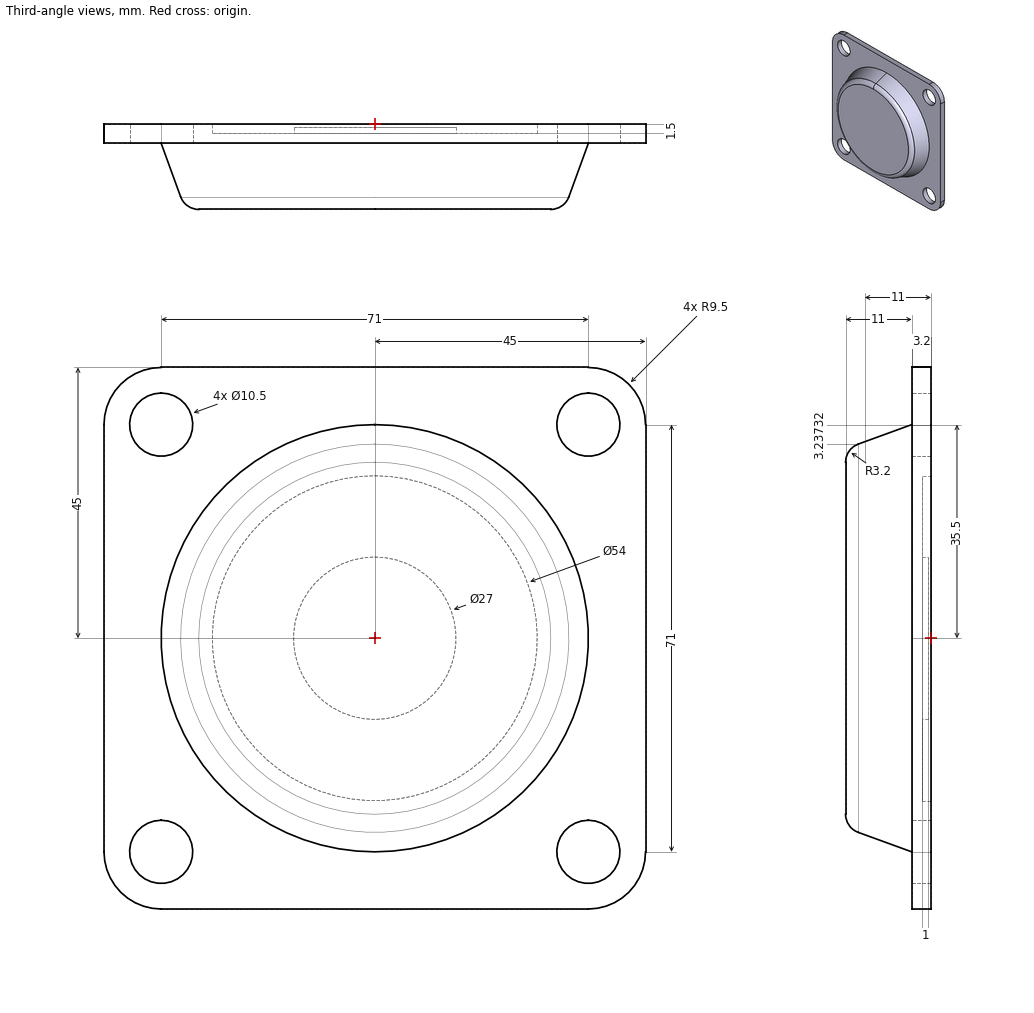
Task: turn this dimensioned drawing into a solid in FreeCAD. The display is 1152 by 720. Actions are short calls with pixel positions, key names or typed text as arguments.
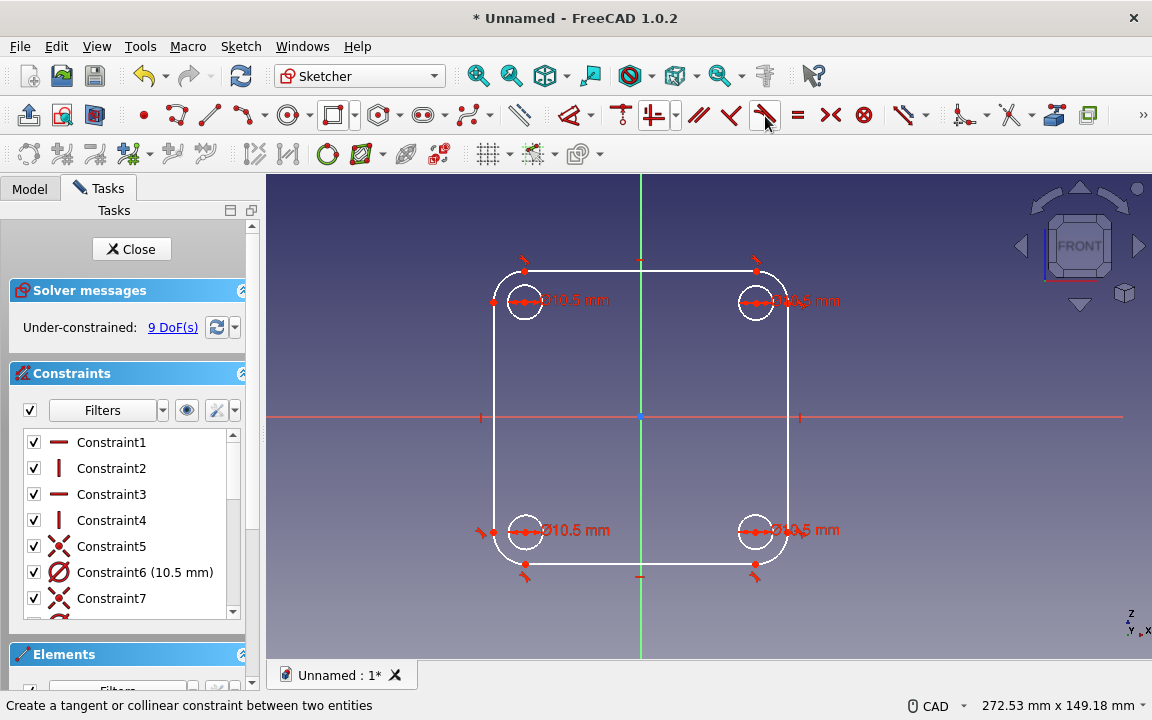
click(494, 463)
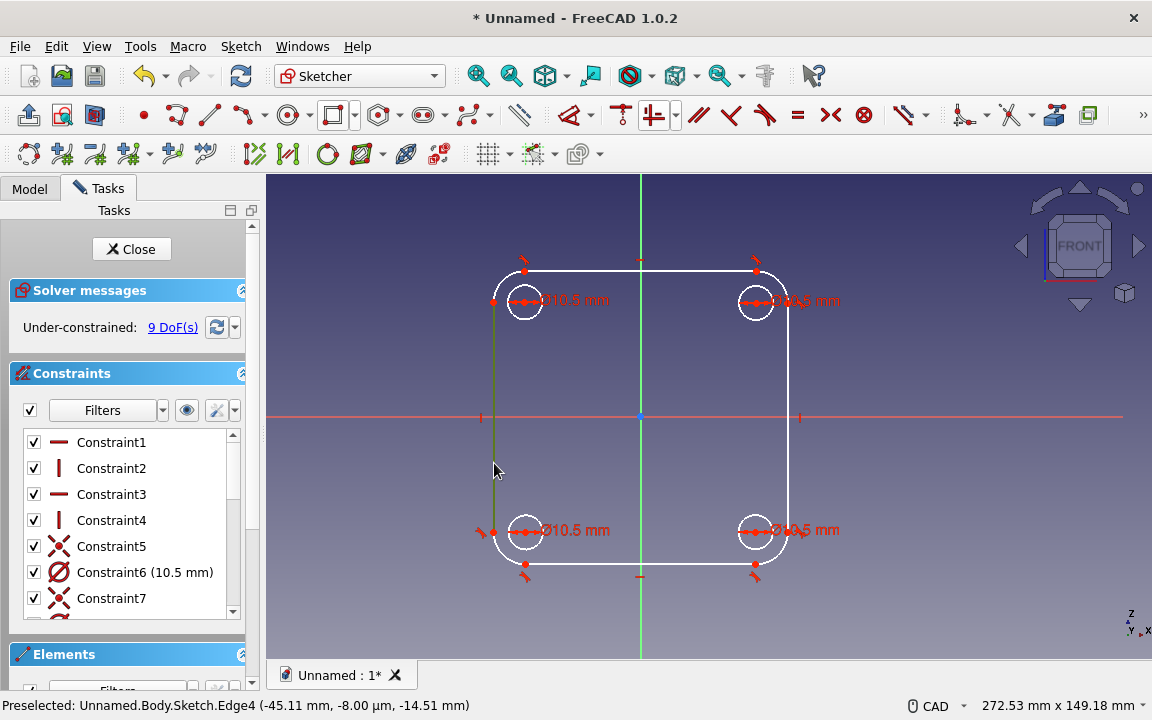
click(511, 275)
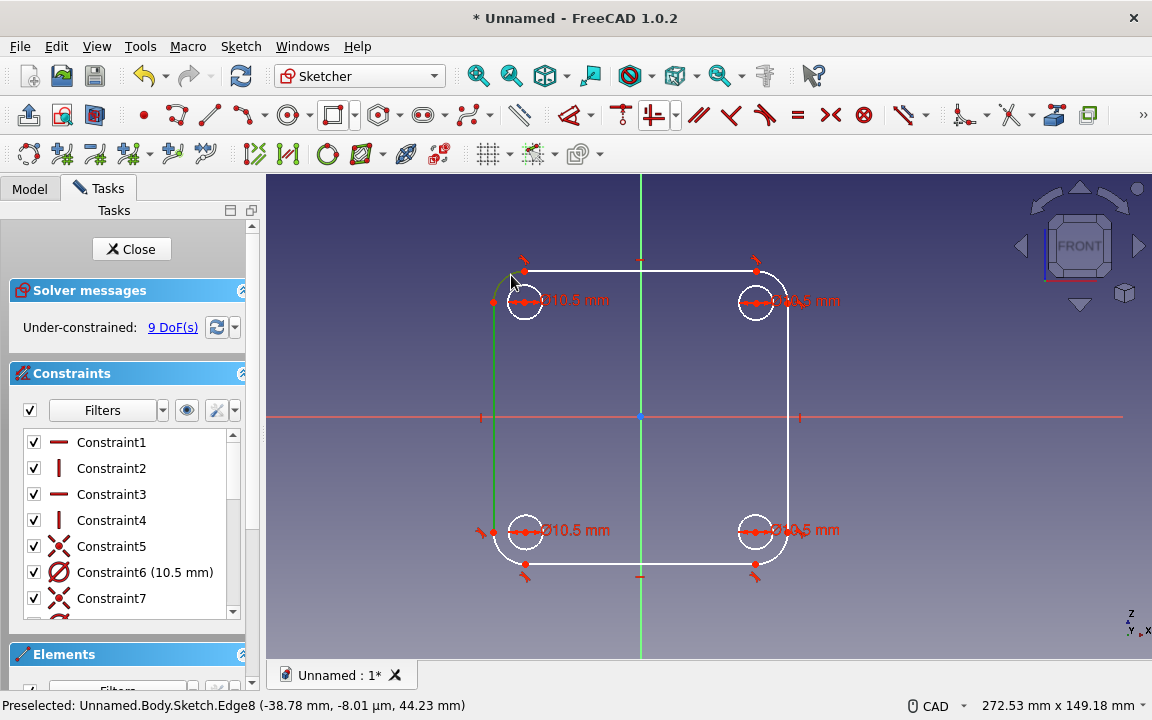
key(t)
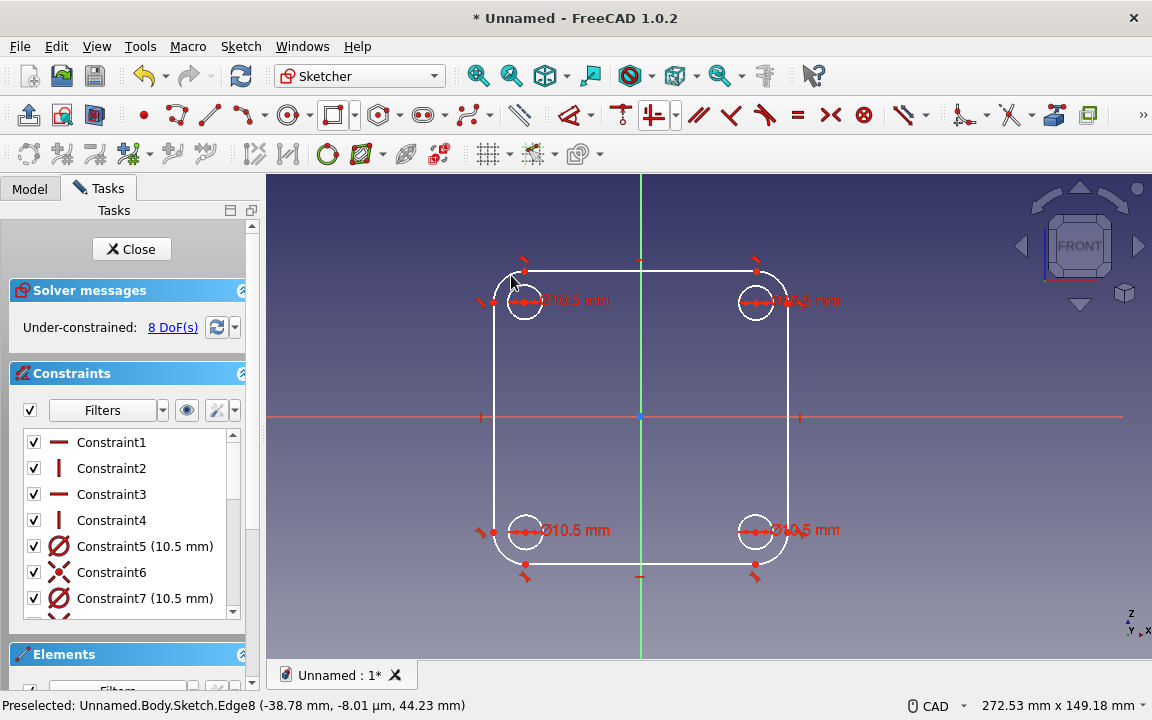
click(784, 289)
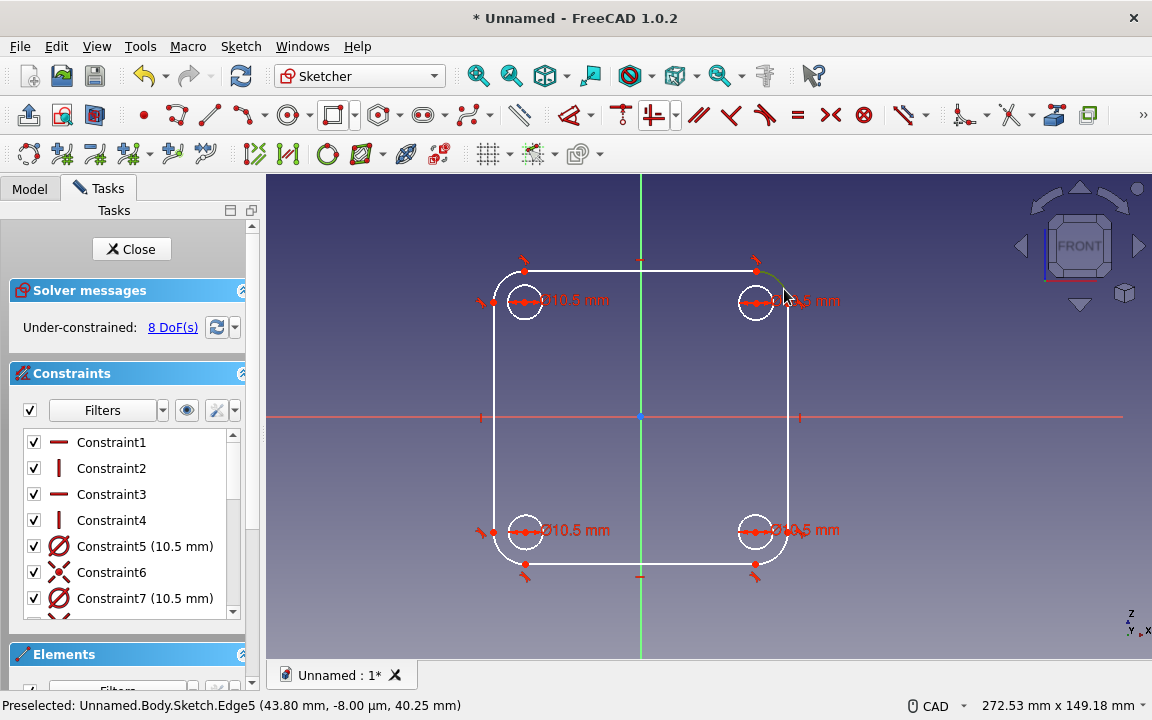
click(770, 561)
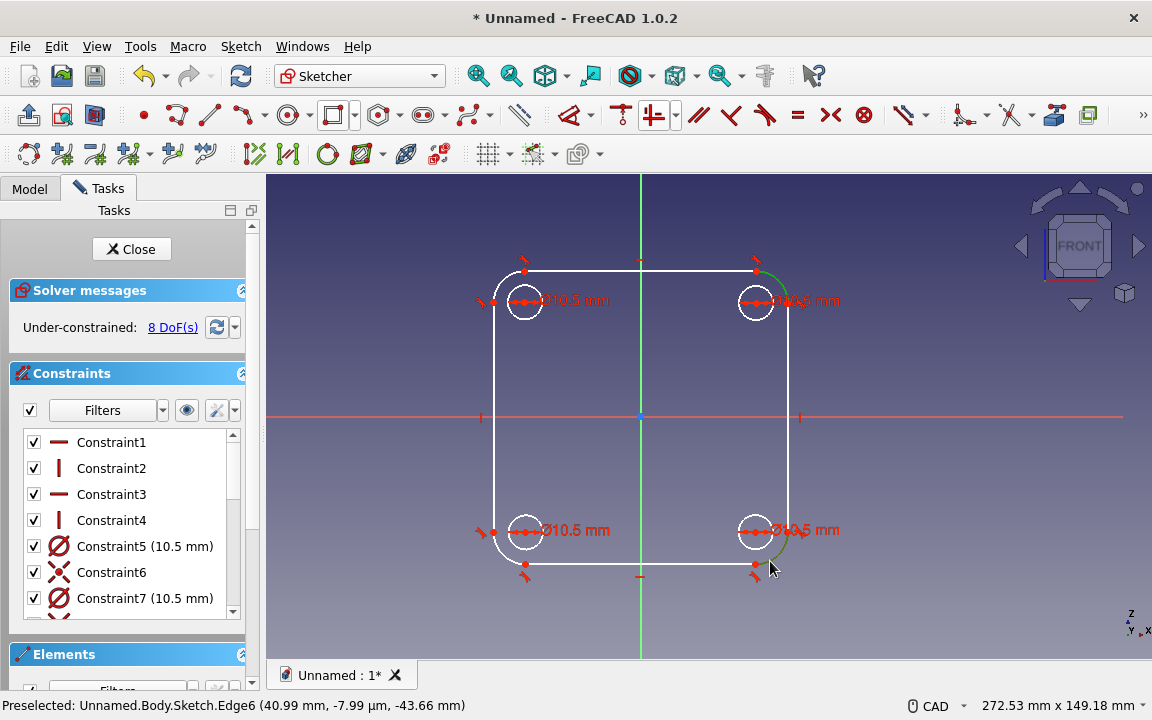
click(497, 547)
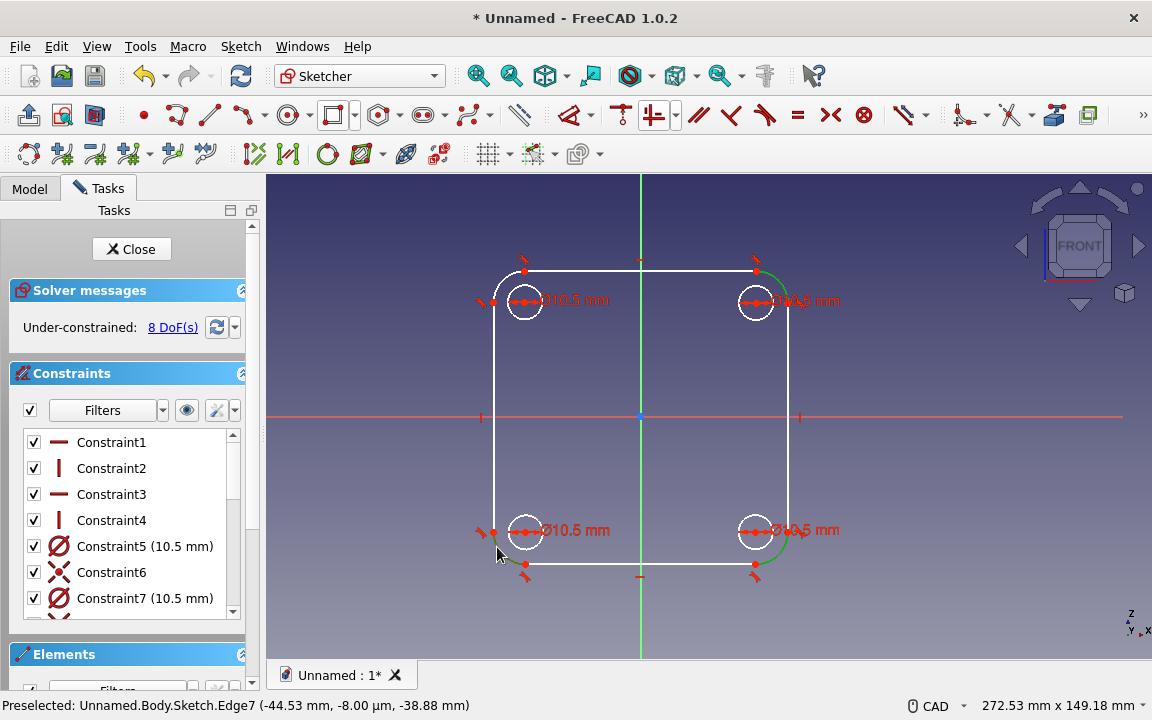
click(511, 275)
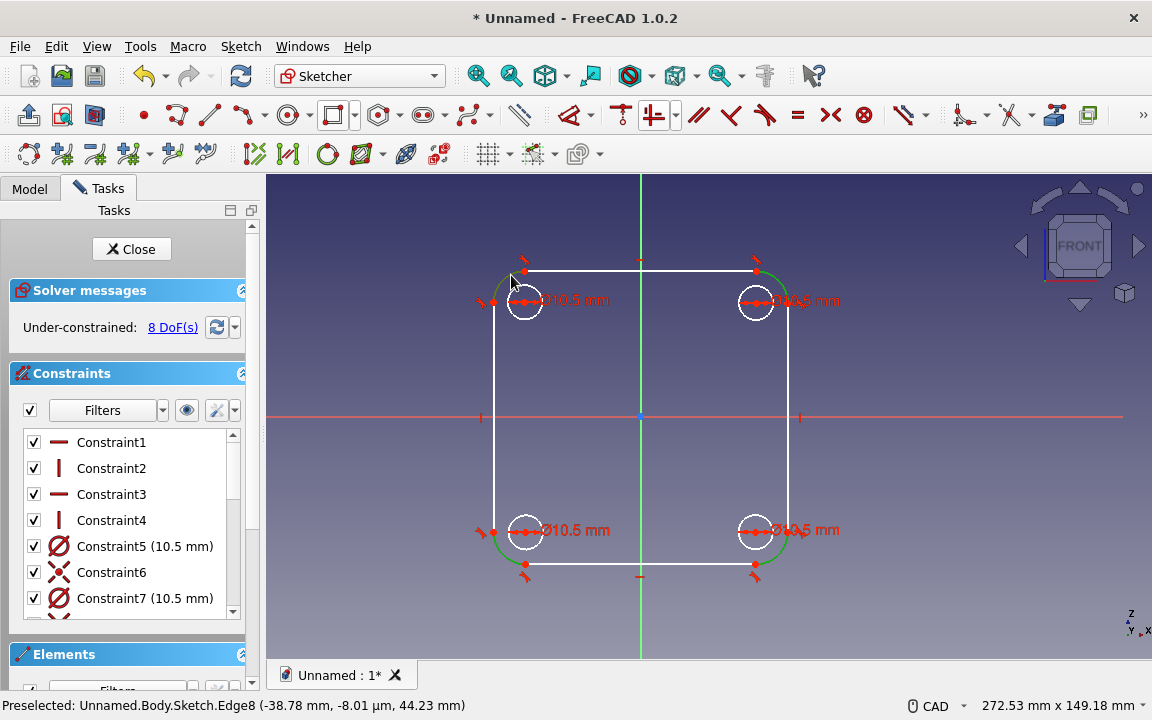
key(e)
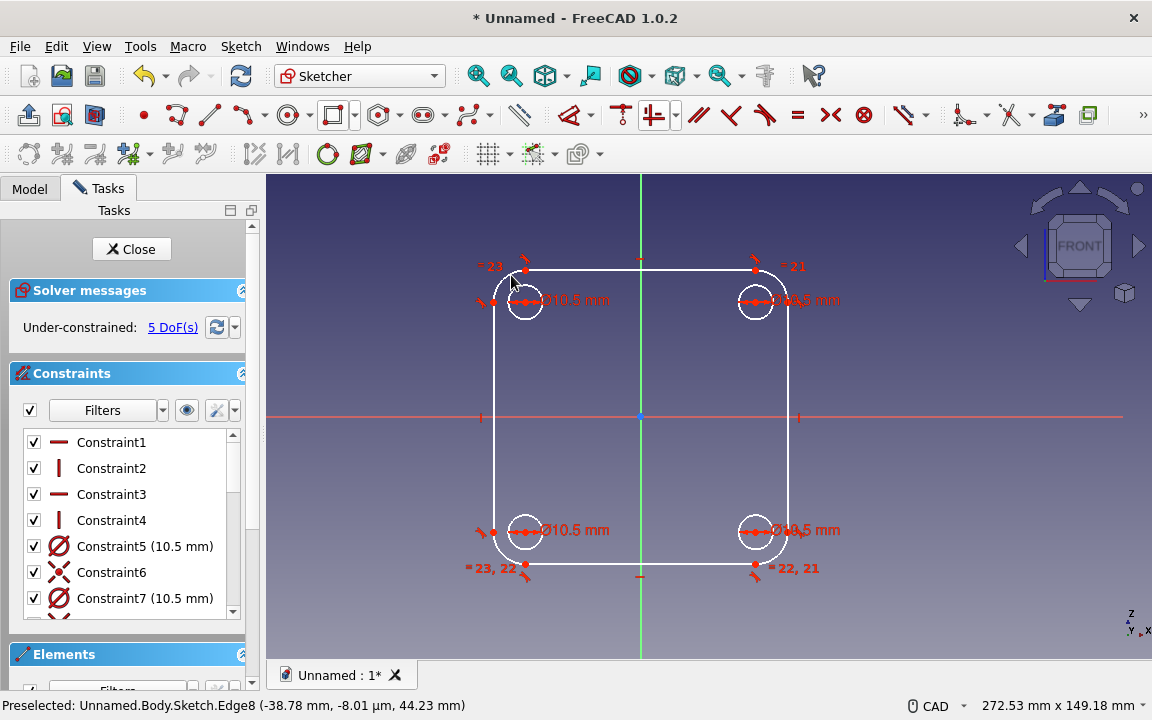
key(d)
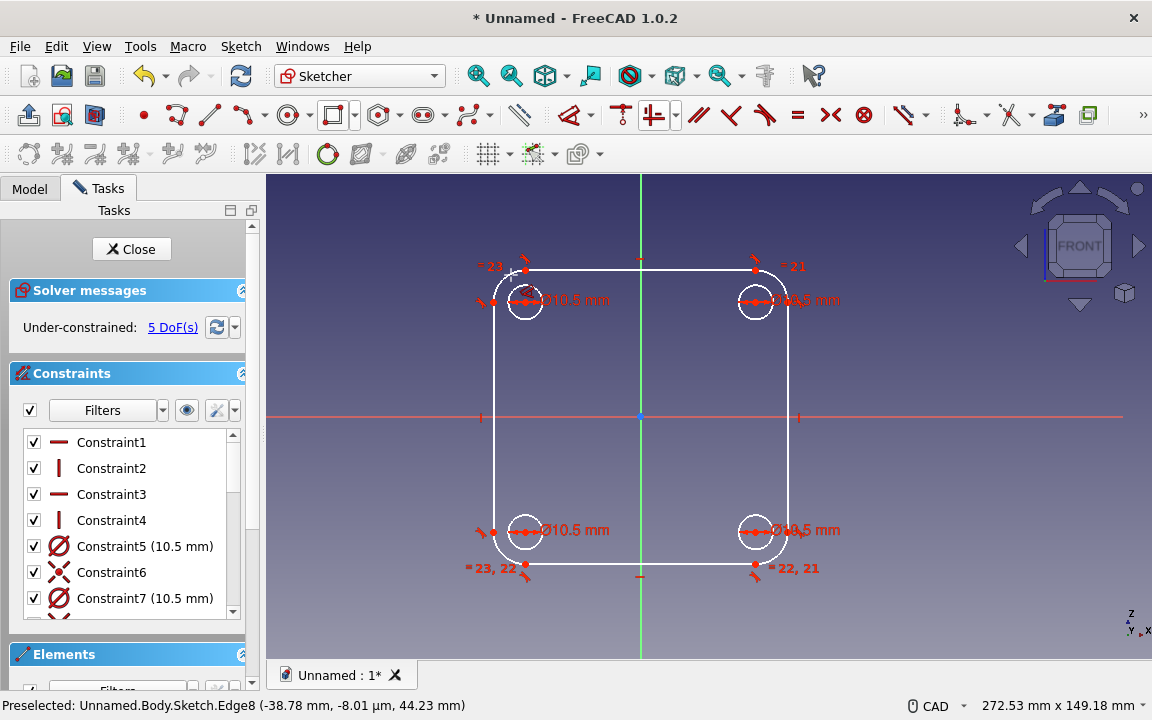
scroll(784, 288, up, 2)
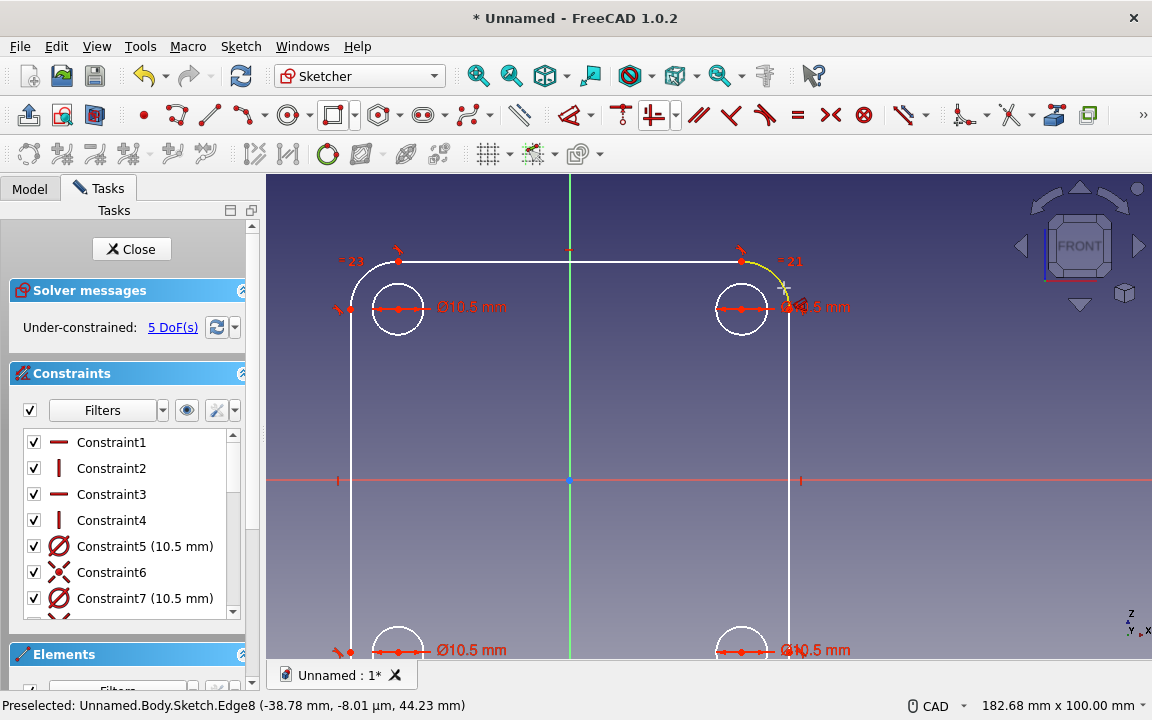
click(784, 288)
click(813, 274)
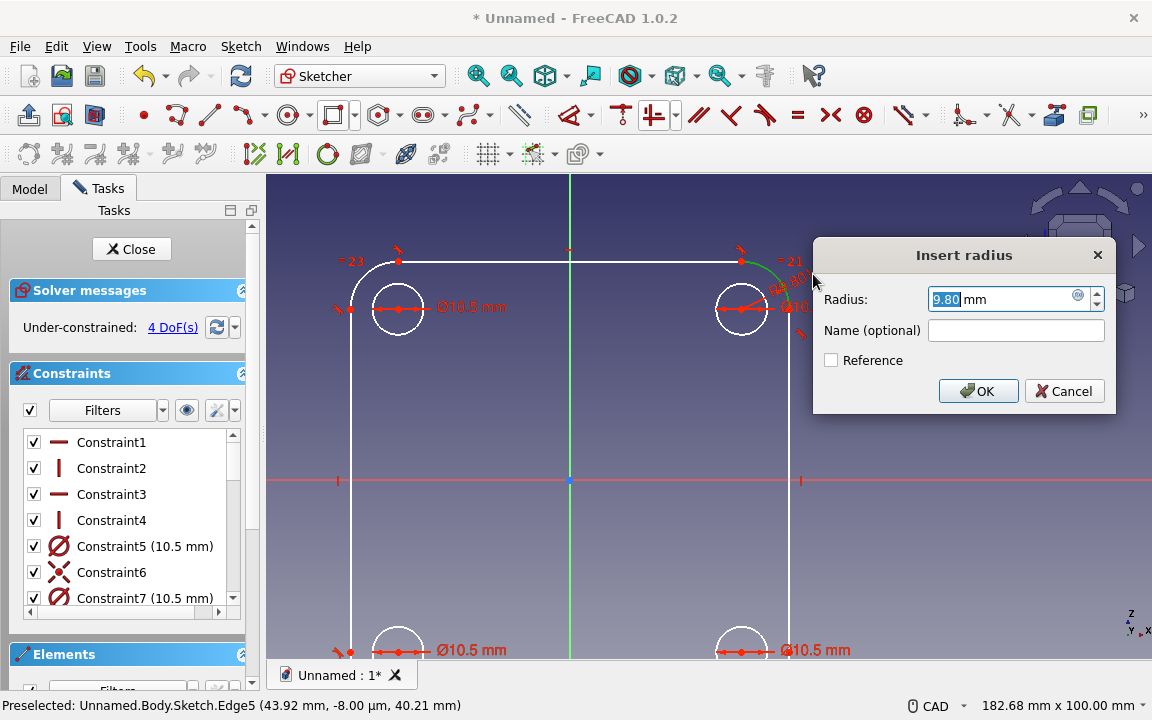
text(9.5)
key(Return)